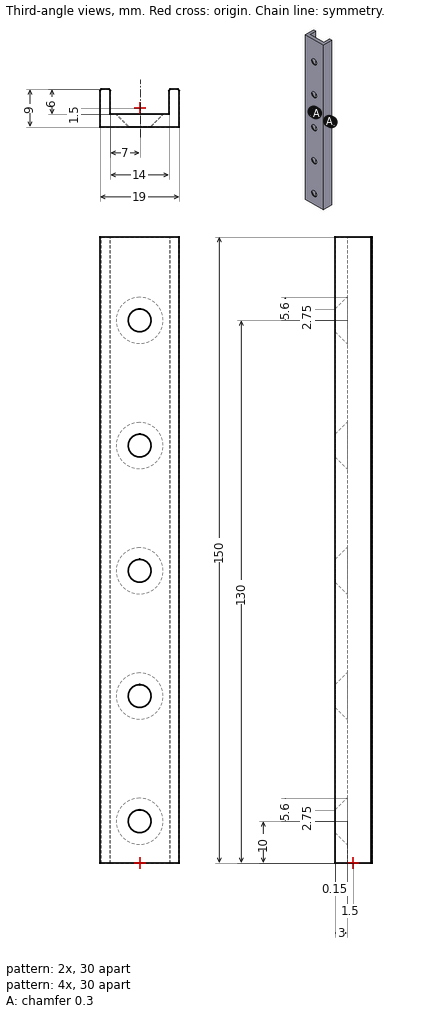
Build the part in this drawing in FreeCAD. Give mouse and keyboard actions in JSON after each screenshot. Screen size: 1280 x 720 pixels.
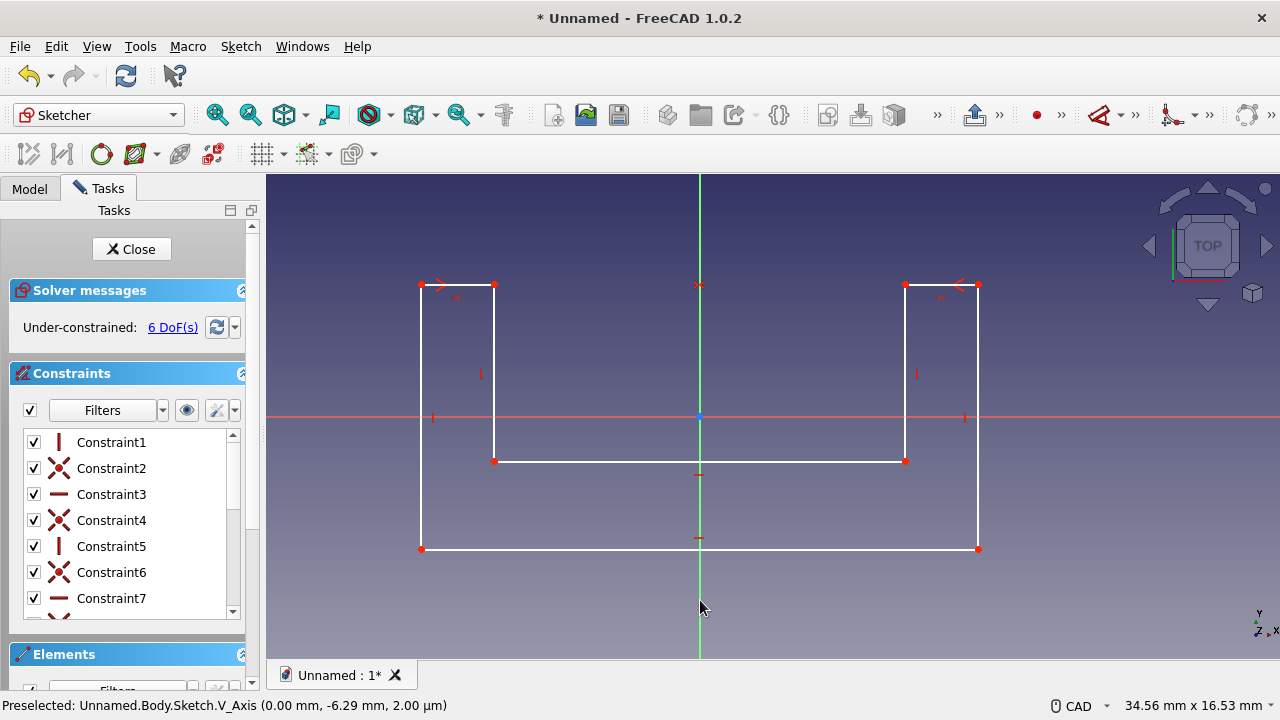
{"action": "left_click", "coordinate": [494, 338]}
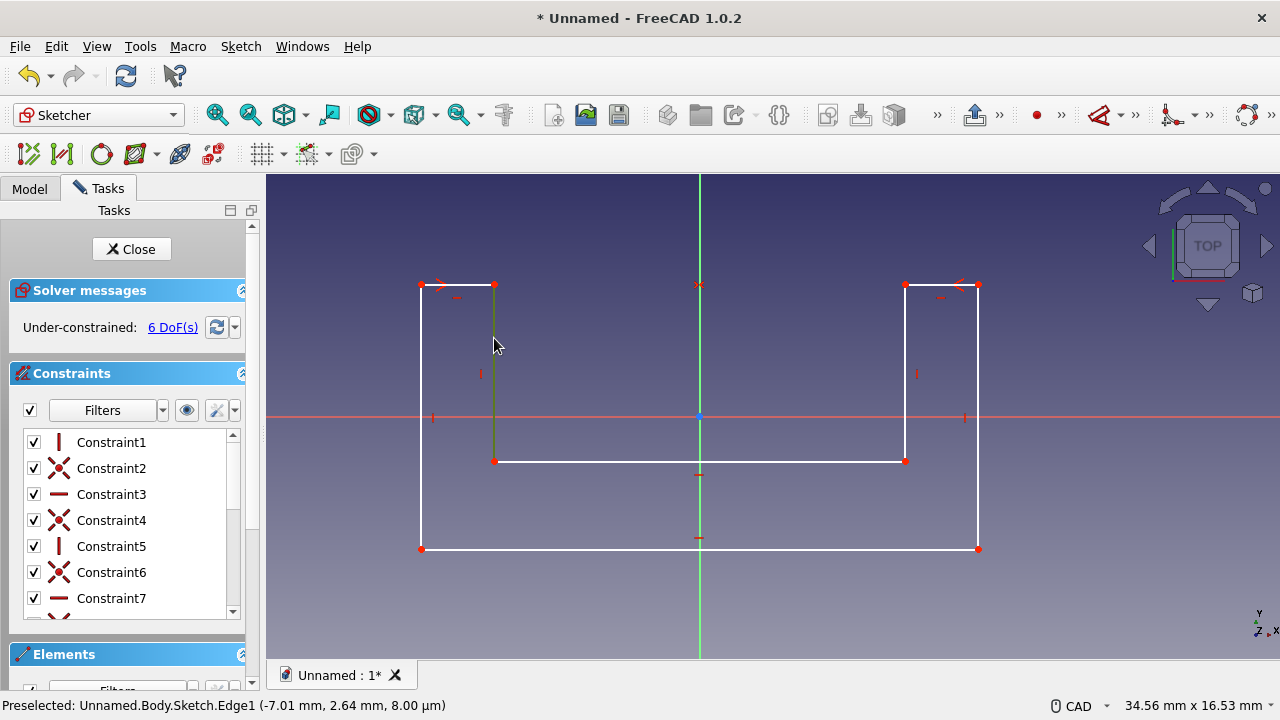
{"action": "key", "text": "i"}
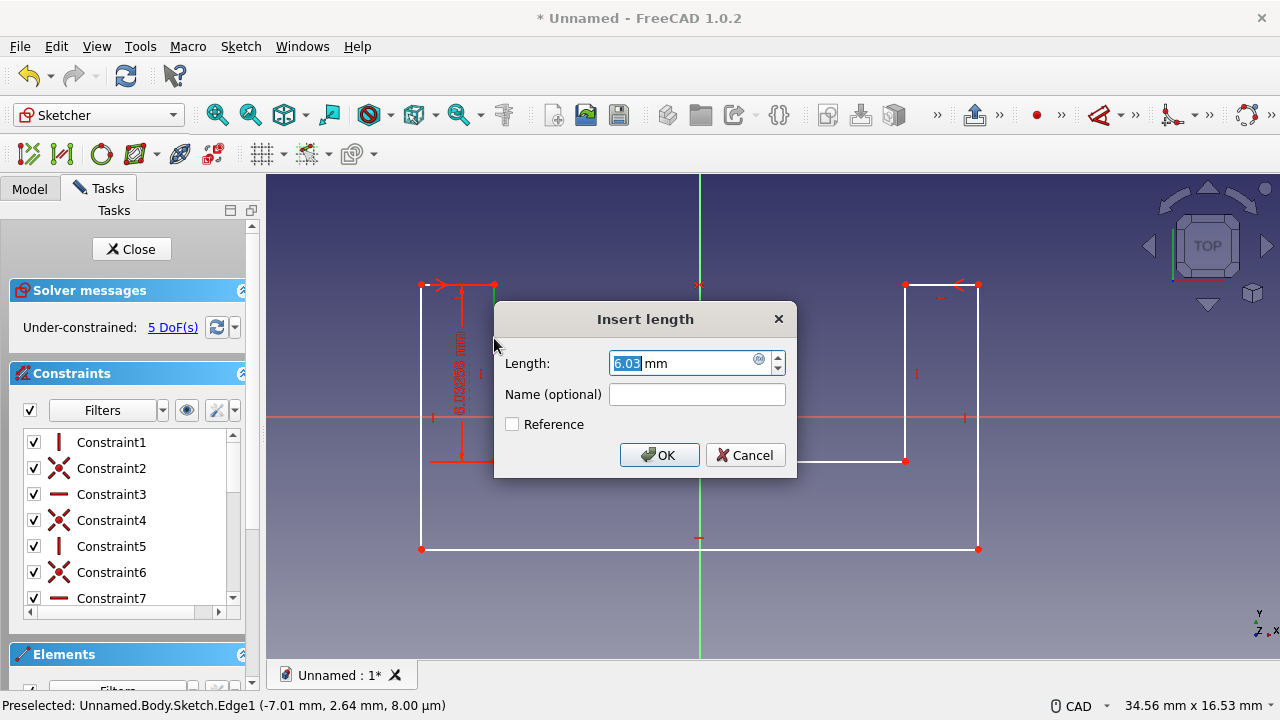
{"action": "type", "text": "6"}
{"action": "key", "text": "Return"}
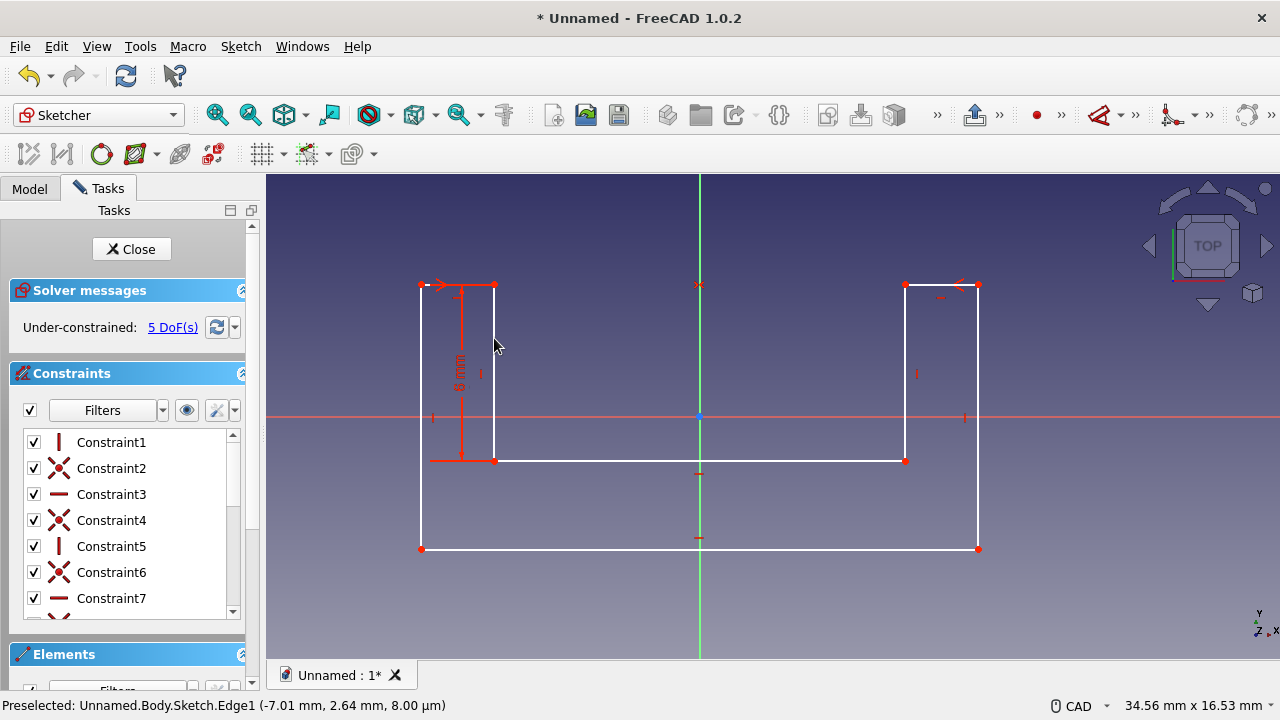
{"action": "left_click", "coordinate": [421, 365]}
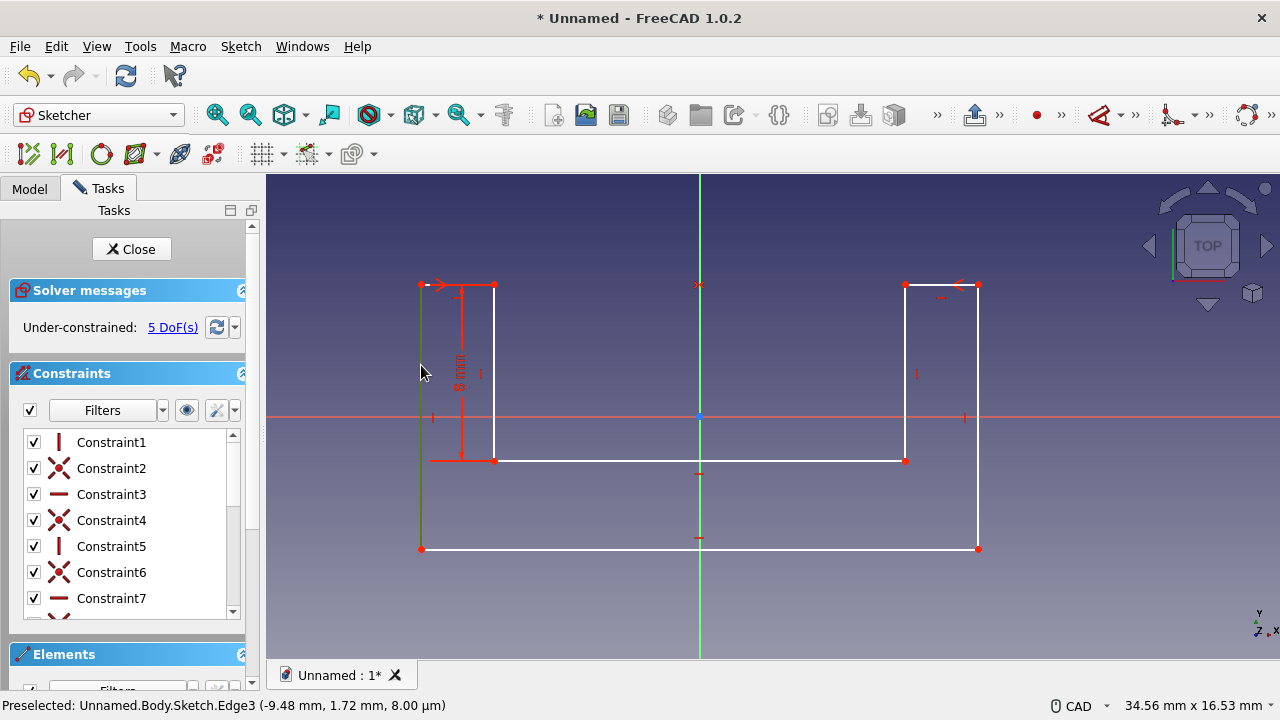
{"action": "left_click", "coordinate": [1120, 116]}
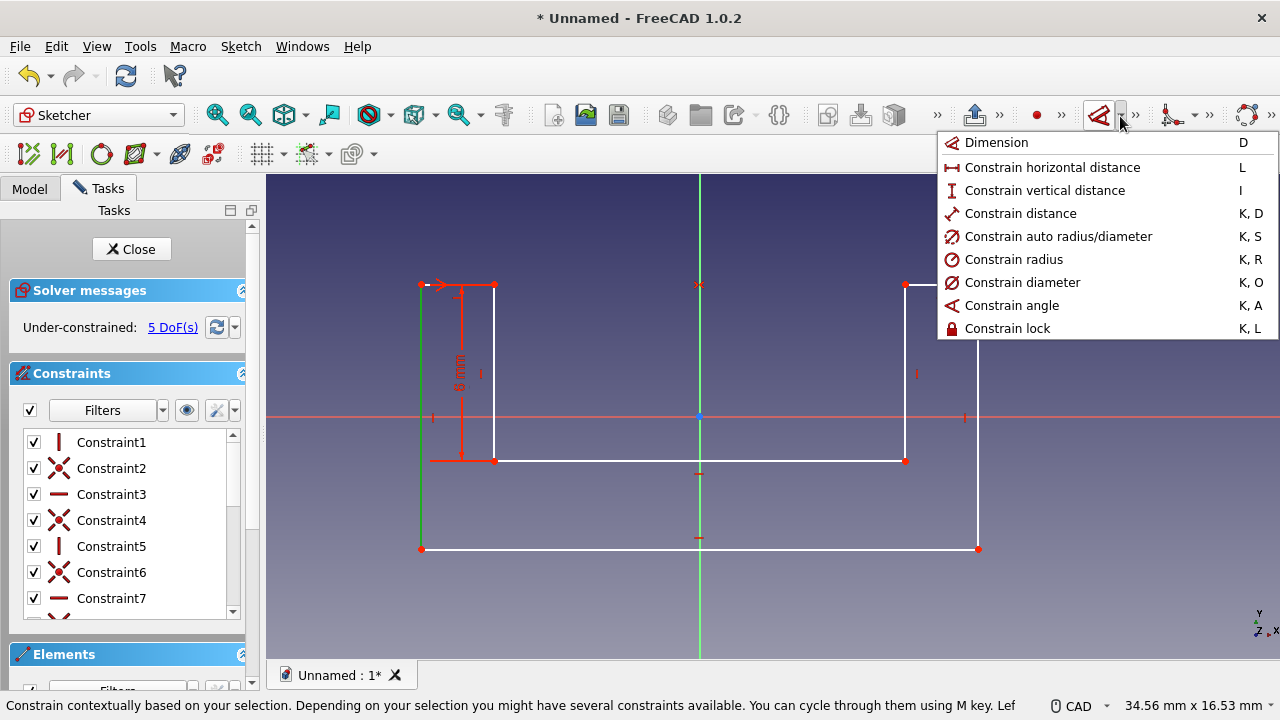
{"action": "left_click", "coordinate": [1108, 190]}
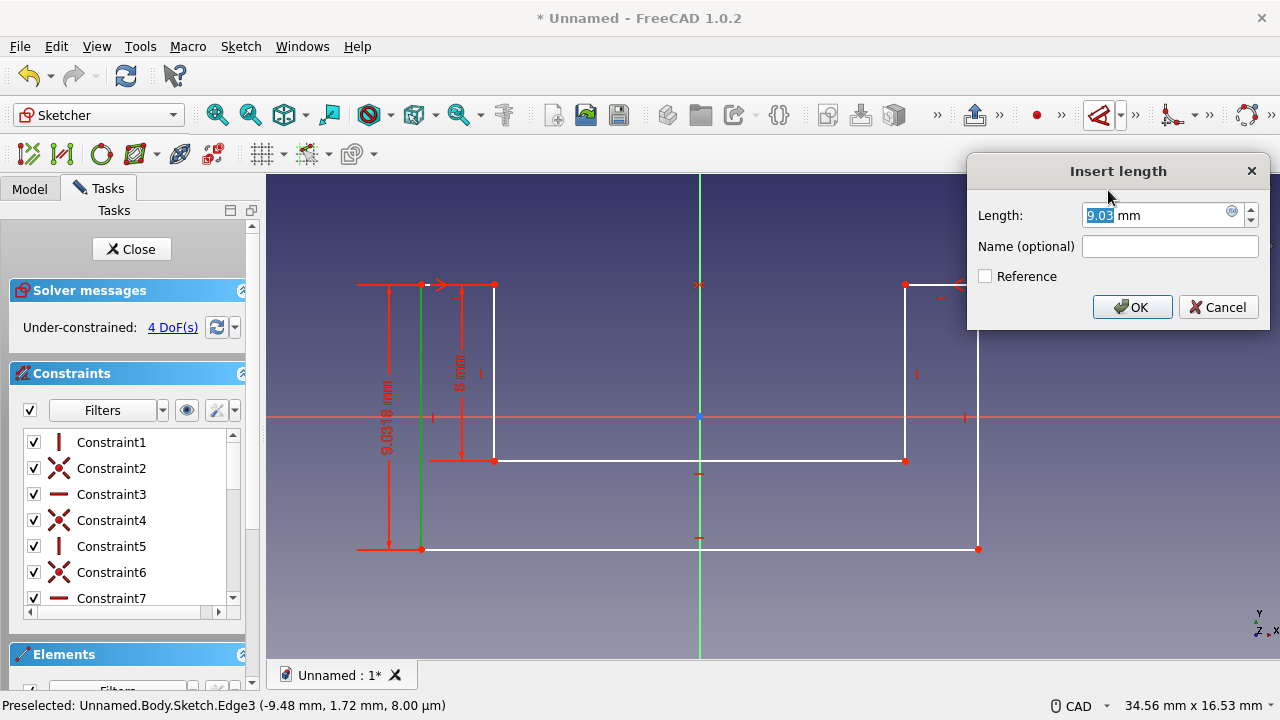
{"action": "type", "text": "9"}
{"action": "key", "text": "Return"}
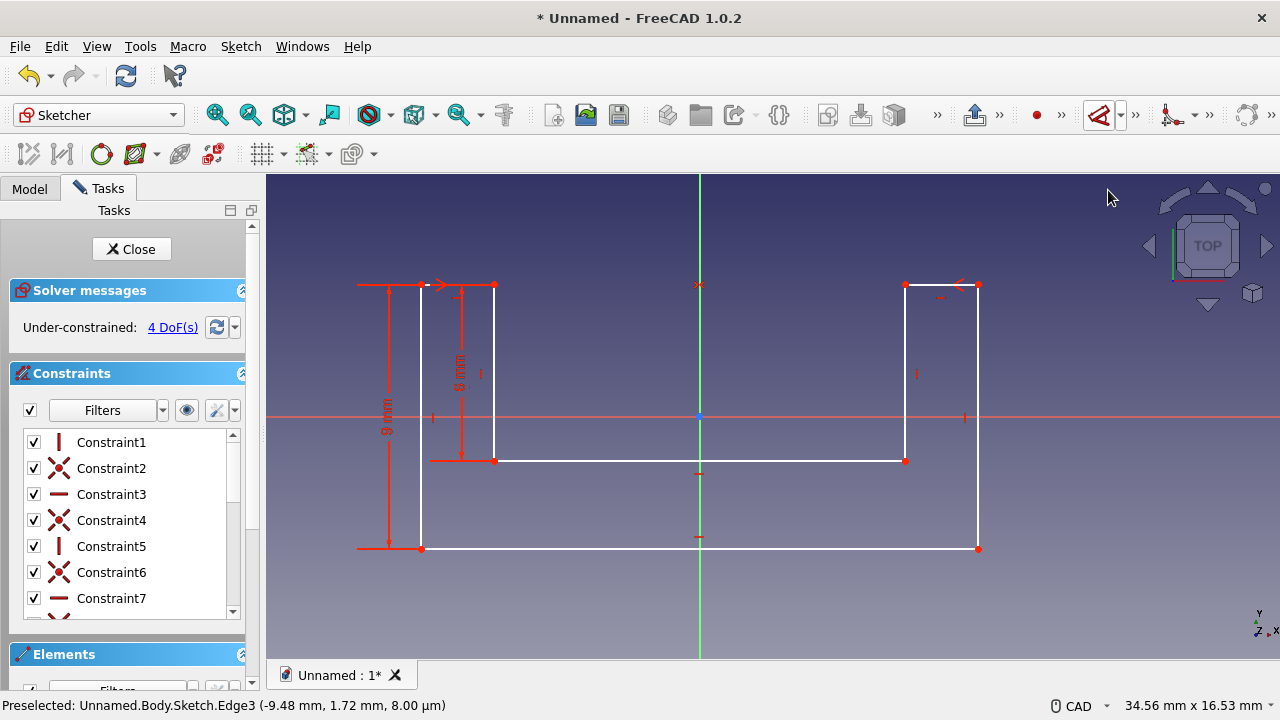
{"action": "left_click", "coordinate": [588, 549]}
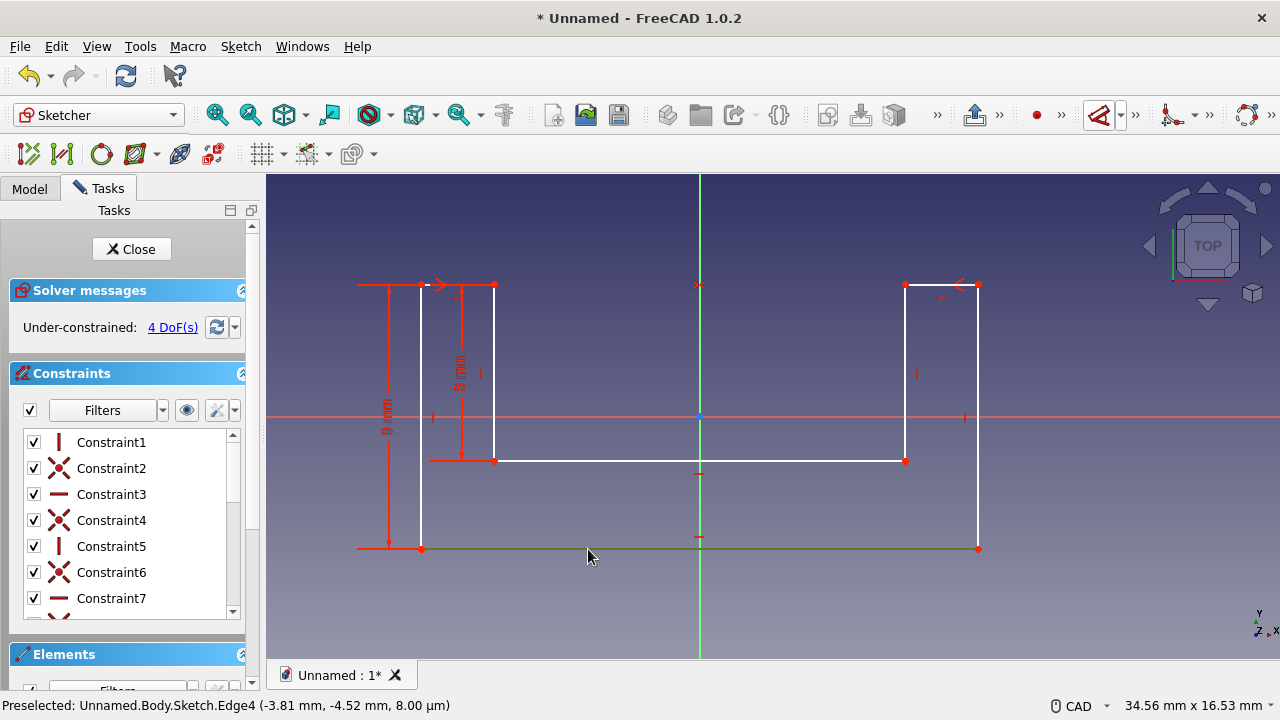
{"action": "key", "text": "l"}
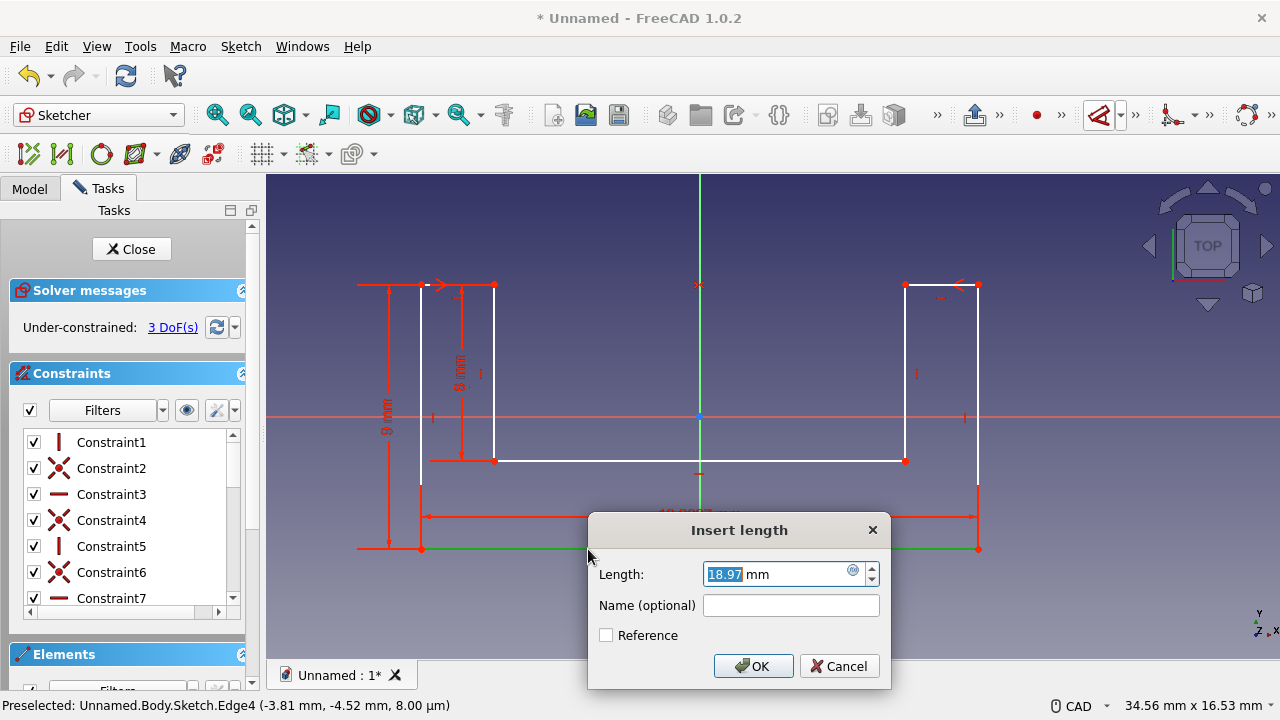
{"action": "type", "text": "19"}
{"action": "key", "text": "Return"}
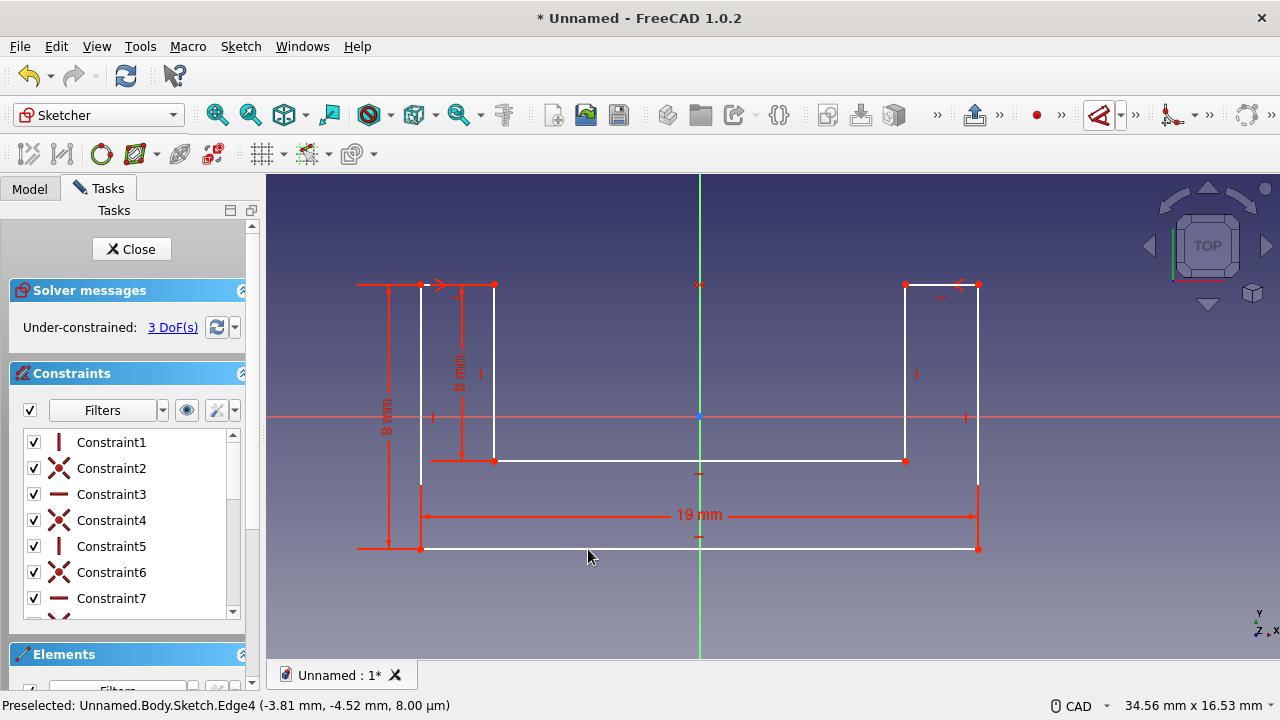
{"action": "left_click", "coordinate": [782, 461]}